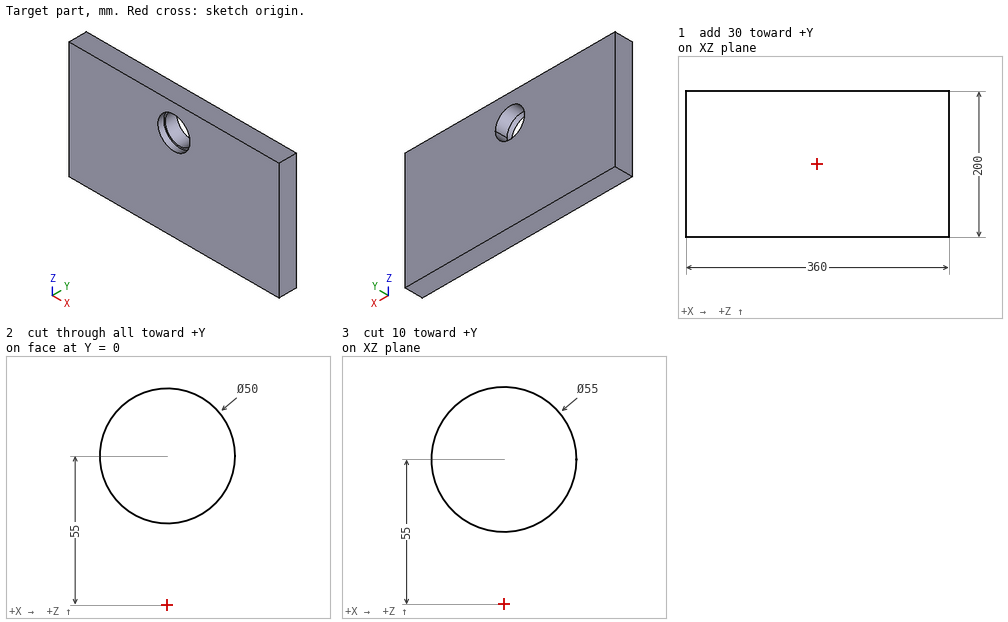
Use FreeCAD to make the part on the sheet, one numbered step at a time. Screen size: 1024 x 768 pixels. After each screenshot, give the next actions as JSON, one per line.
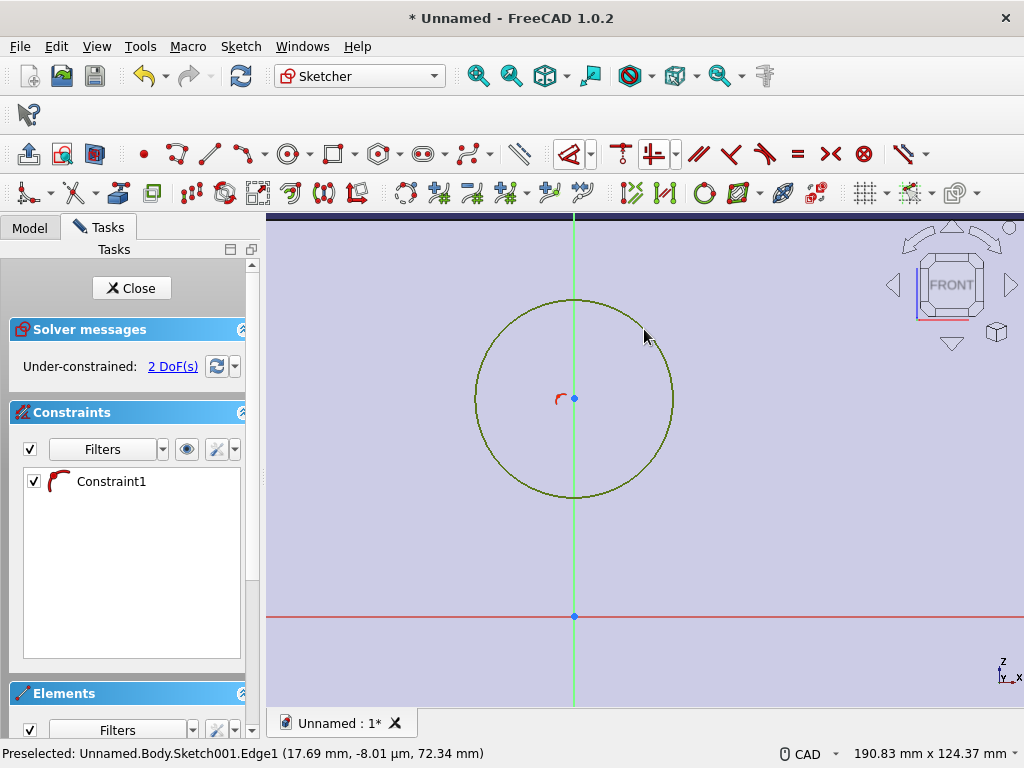
{"action": "key", "text": "k o"}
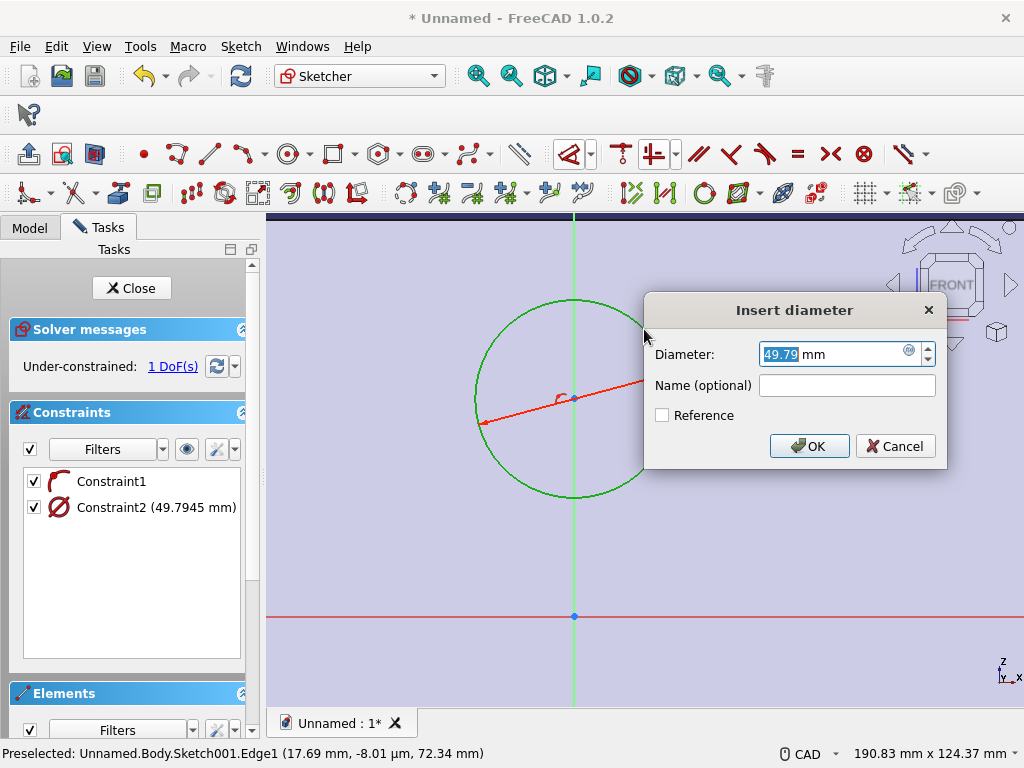
{"action": "type", "text": "50"}
{"action": "key", "text": "Return"}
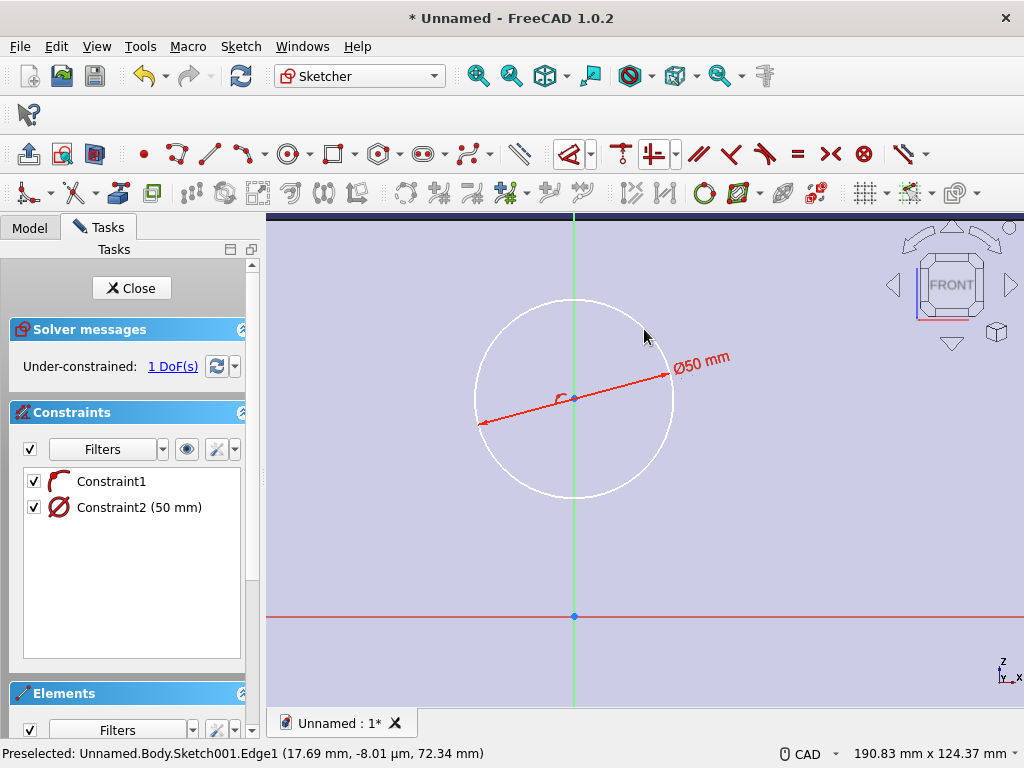
{"action": "left_click", "coordinate": [574, 399]}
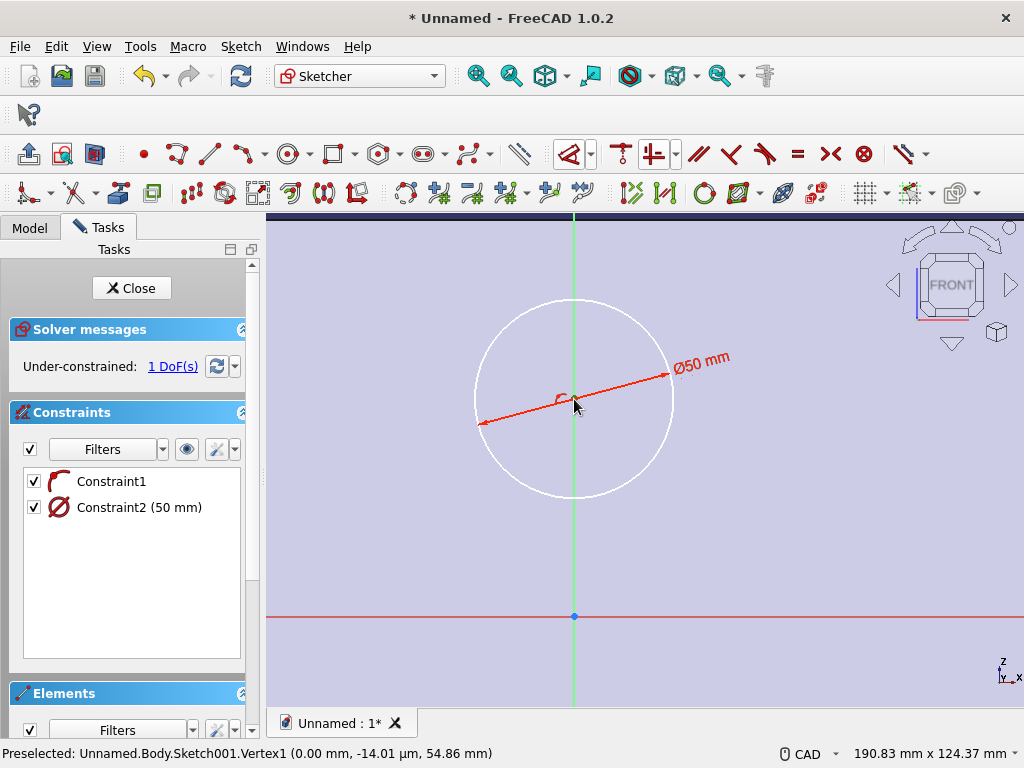
{"action": "key", "text": "i"}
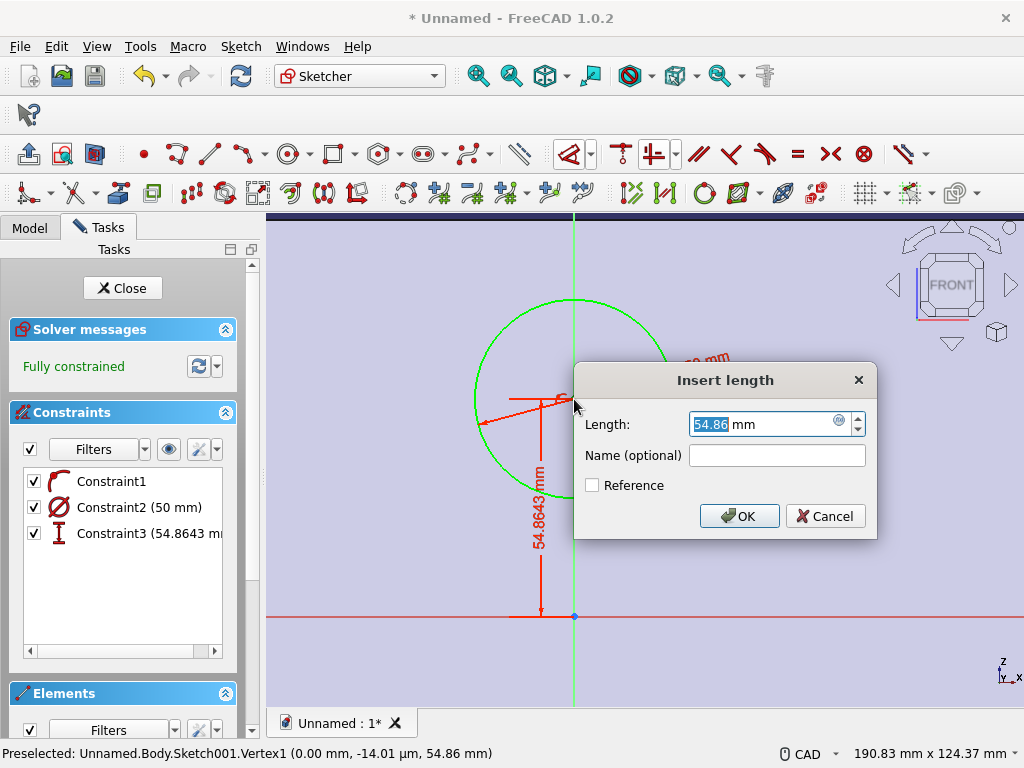
{"action": "type", "text": "55"}
{"action": "key", "text": "Return"}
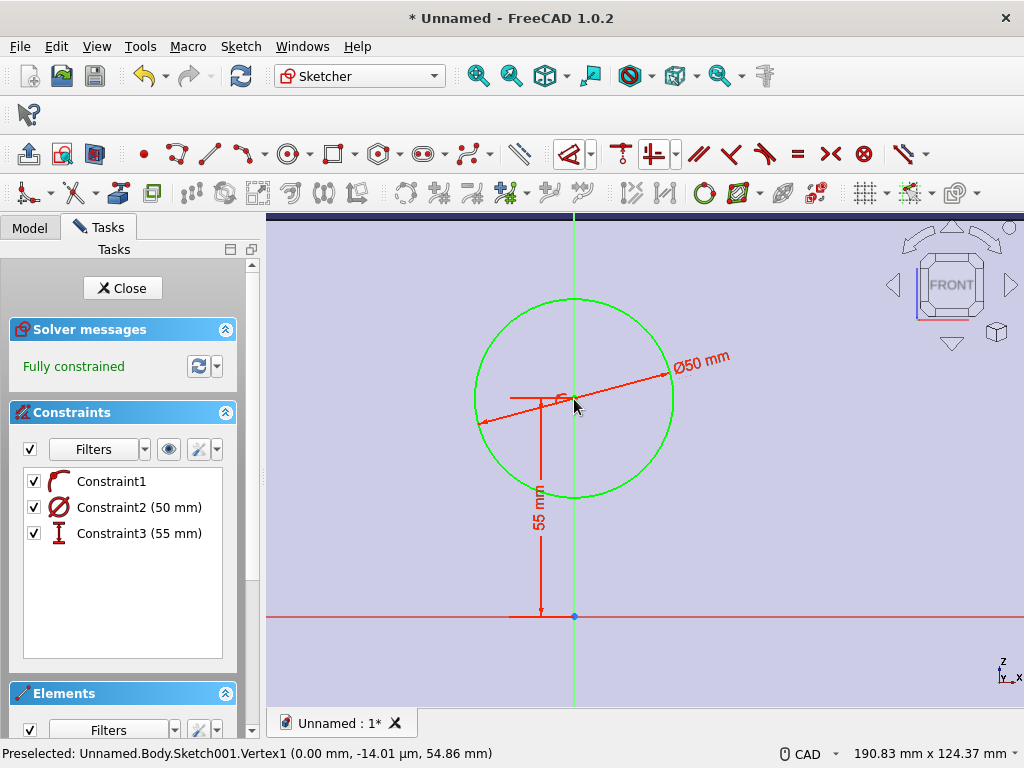
{"action": "left_click", "coordinate": [123, 288]}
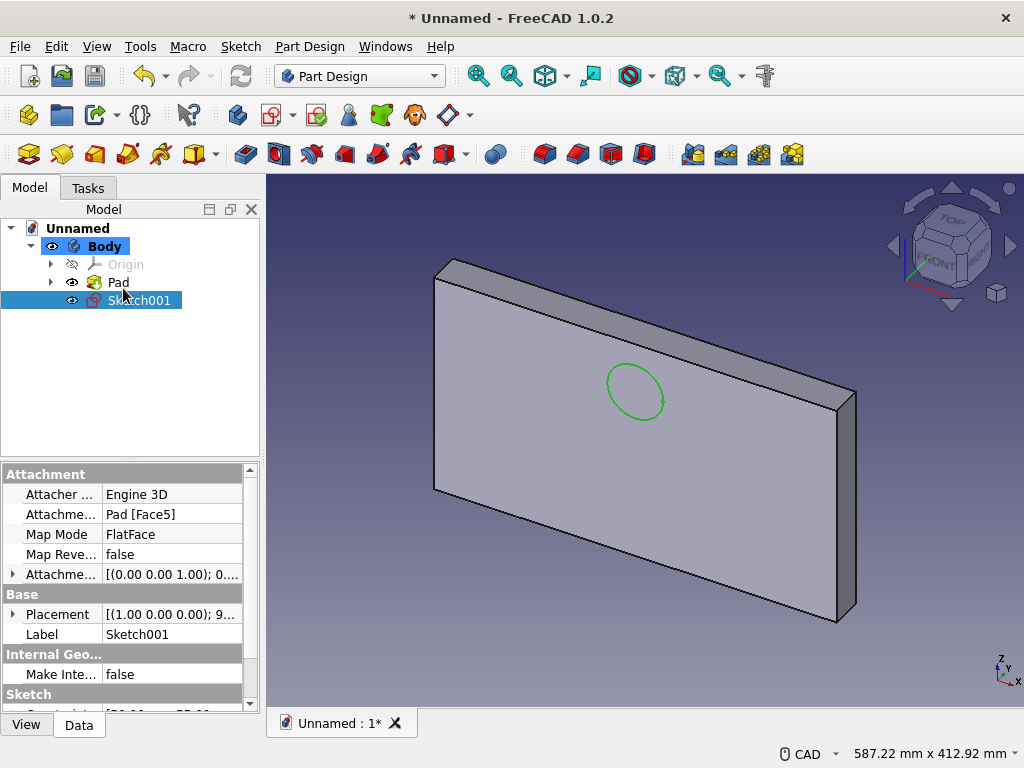
{"action": "left_click", "coordinate": [246, 154]}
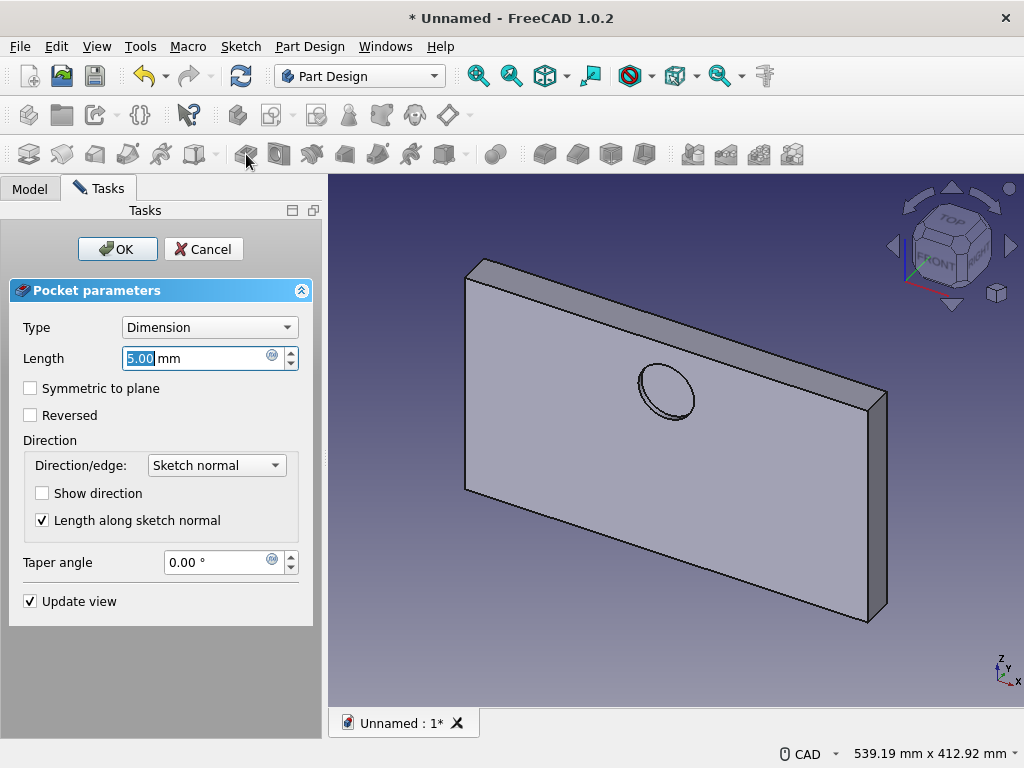
{"action": "left_click", "coordinate": [210, 328]}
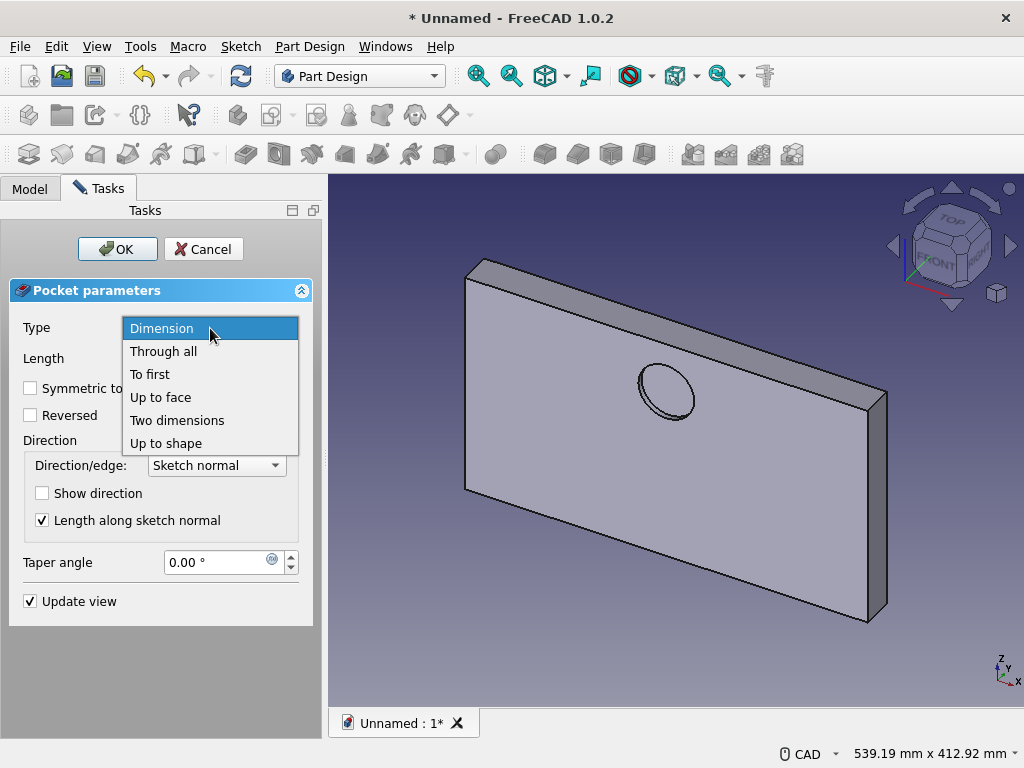
{"action": "left_click", "coordinate": [208, 352]}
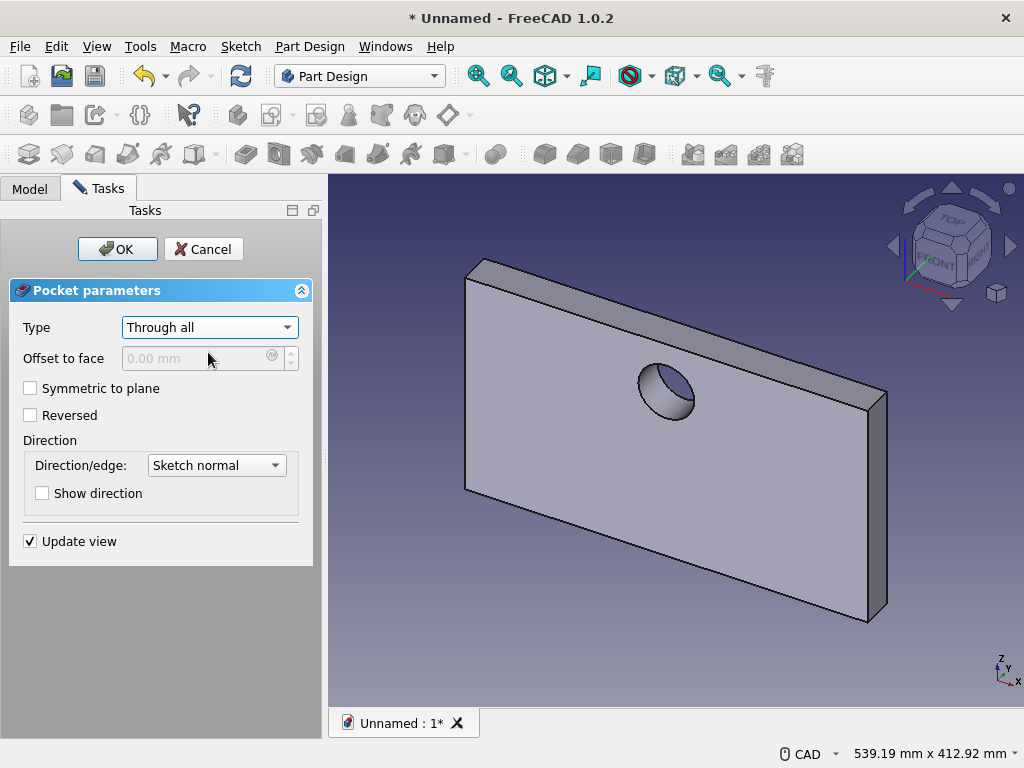
{"action": "left_click", "coordinate": [118, 249]}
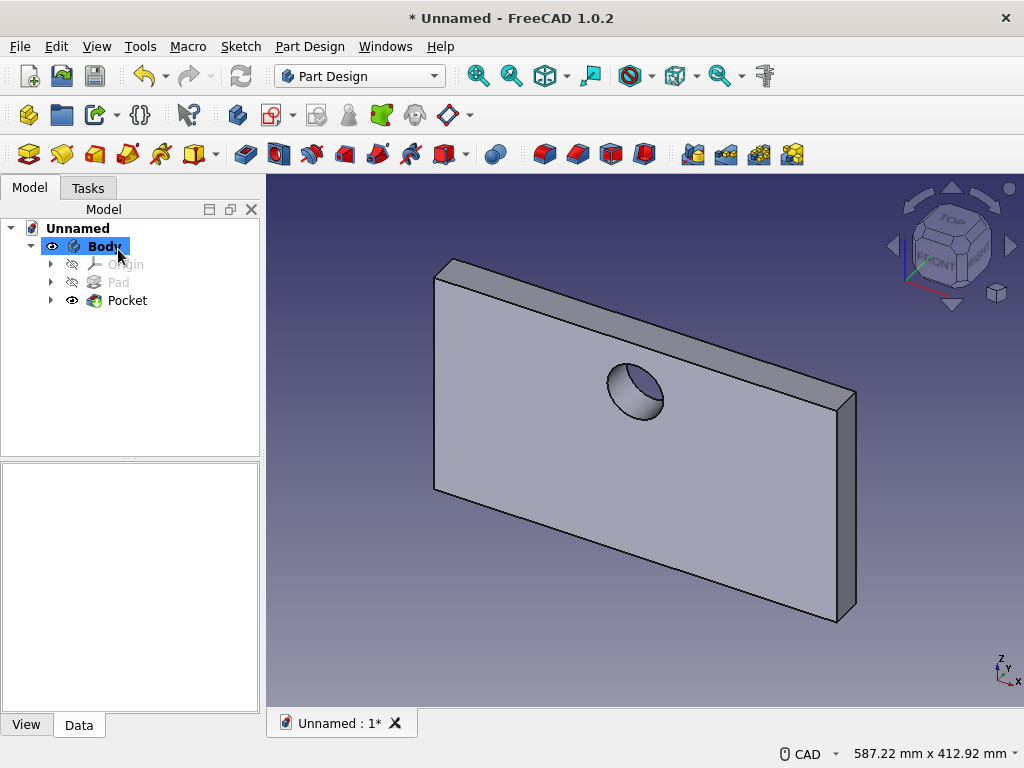
{"action": "left_click", "coordinate": [270, 116]}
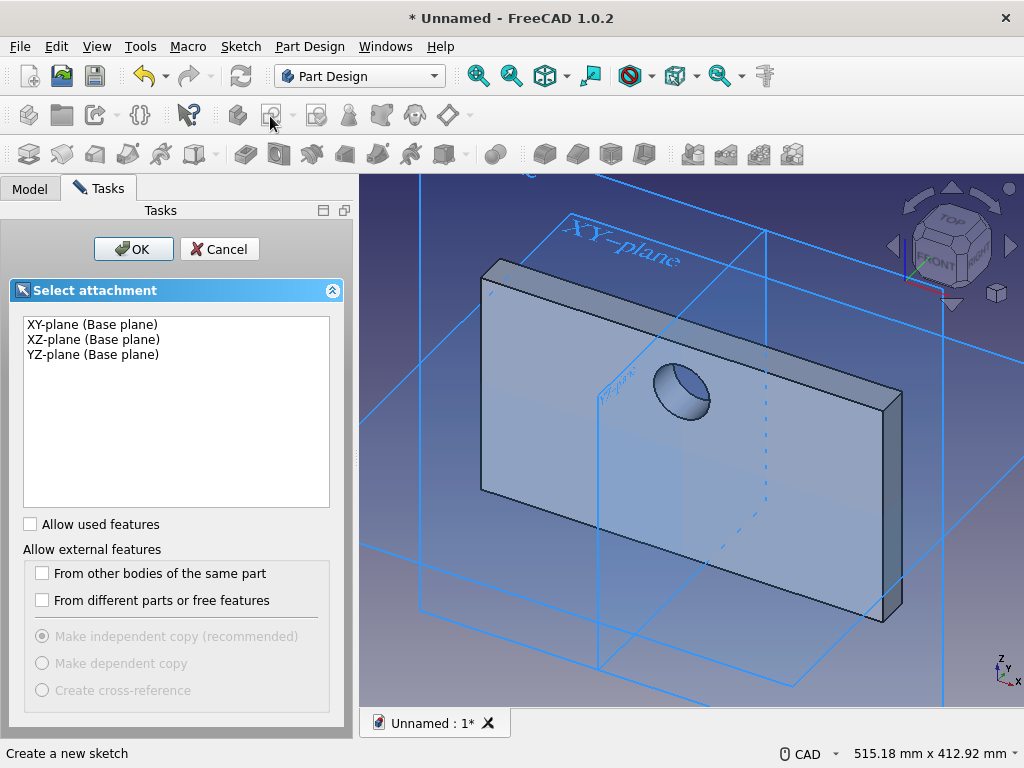
{"action": "left_click", "coordinate": [84, 340]}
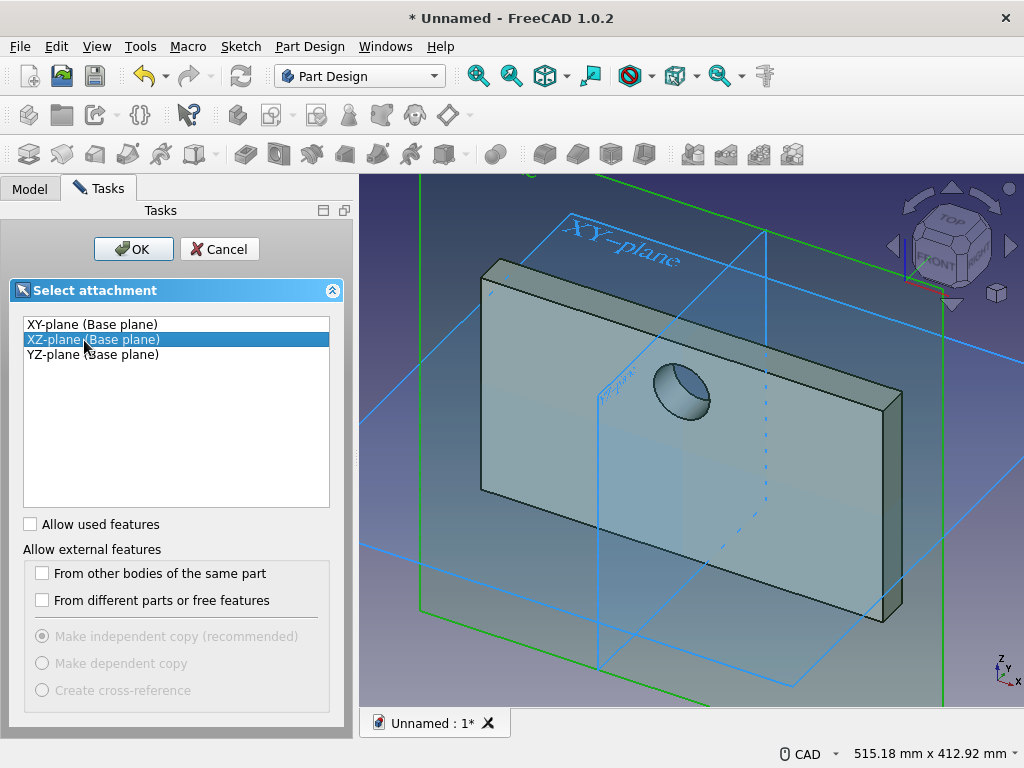
{"action": "left_click", "coordinate": [134, 249]}